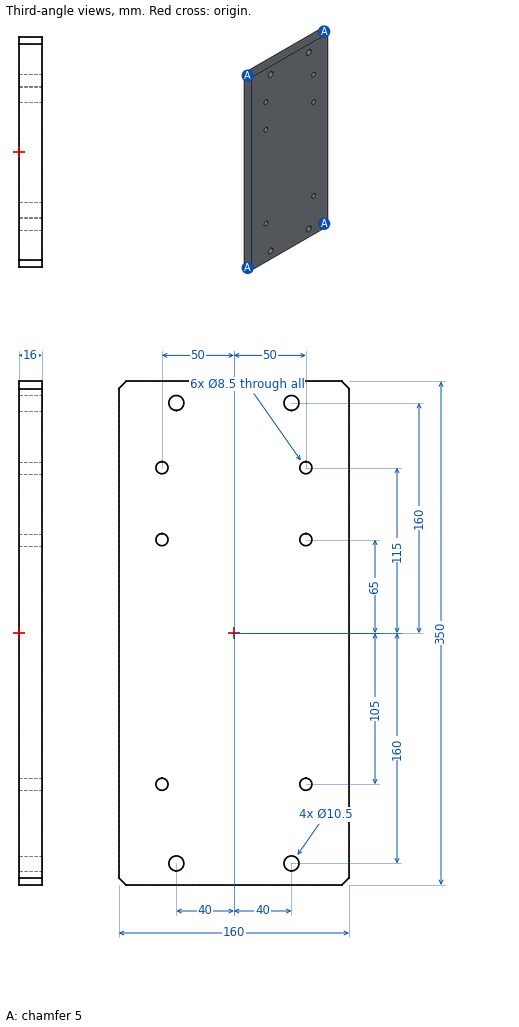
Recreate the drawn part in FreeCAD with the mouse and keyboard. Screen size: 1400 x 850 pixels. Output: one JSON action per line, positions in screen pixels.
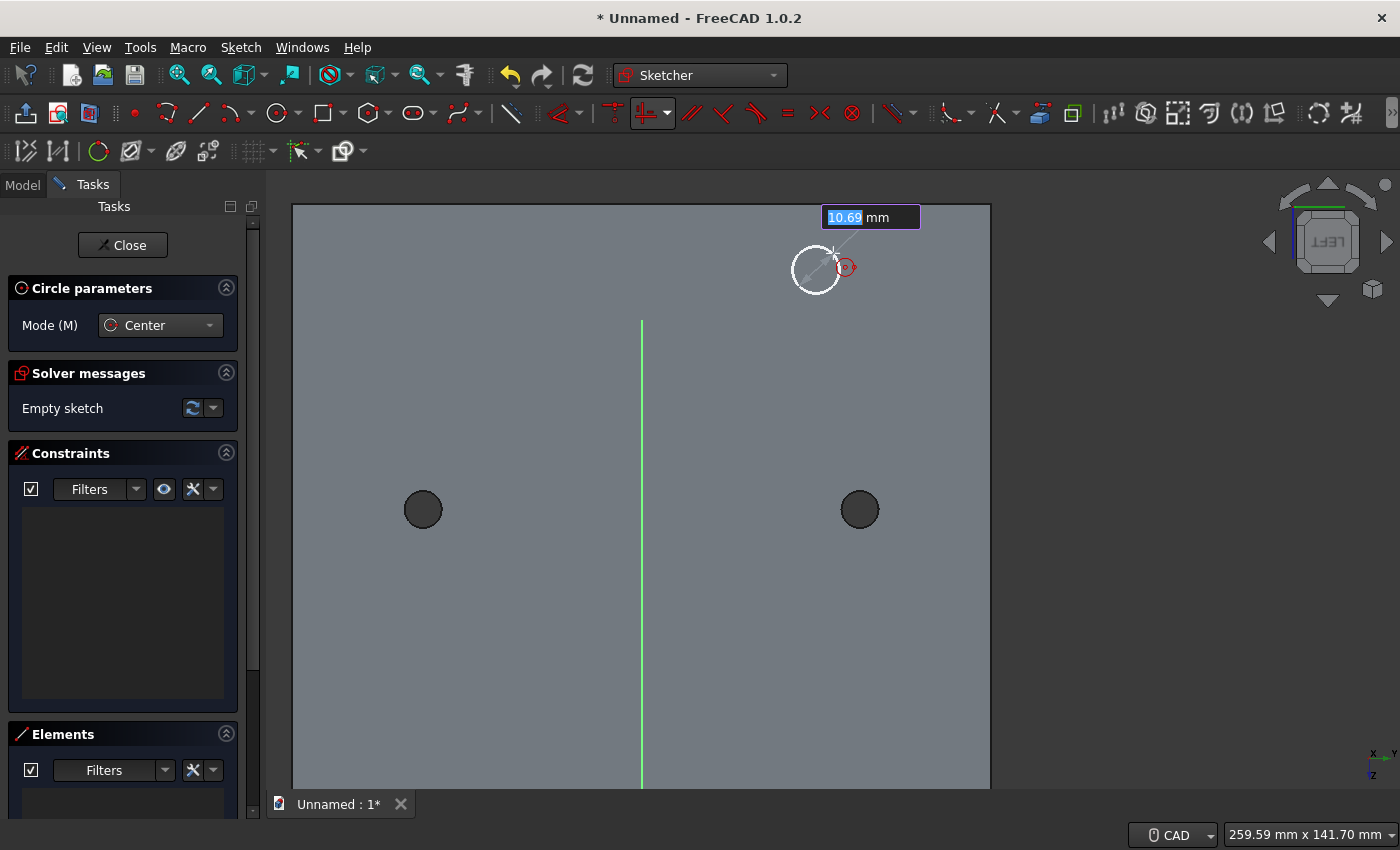
{"action": "type", "text": "10.5"}
{"action": "key", "text": "Return"}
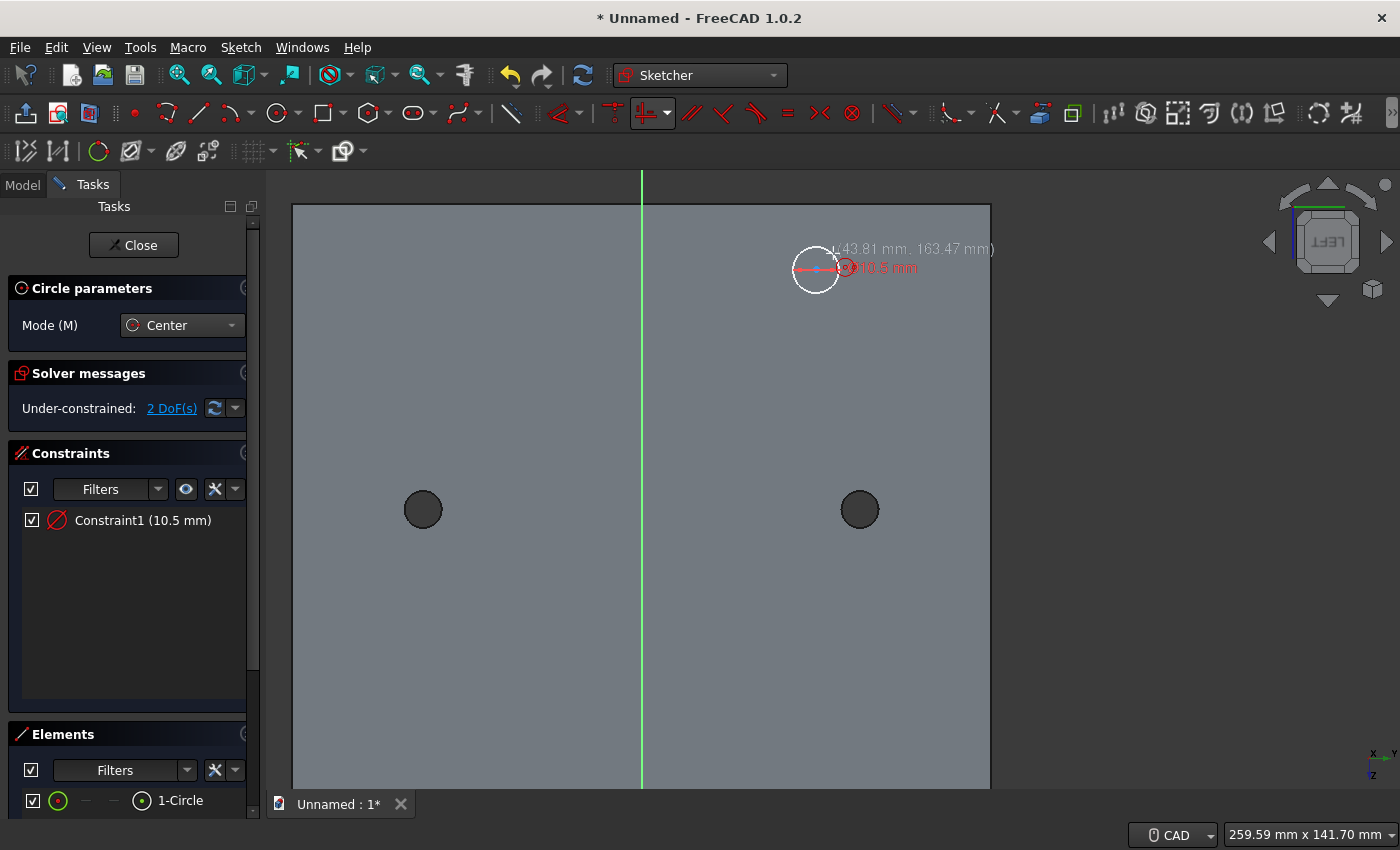
{"action": "left_click", "coordinate": [467, 269]}
{"action": "mouse_move", "coordinate": [483, 253]}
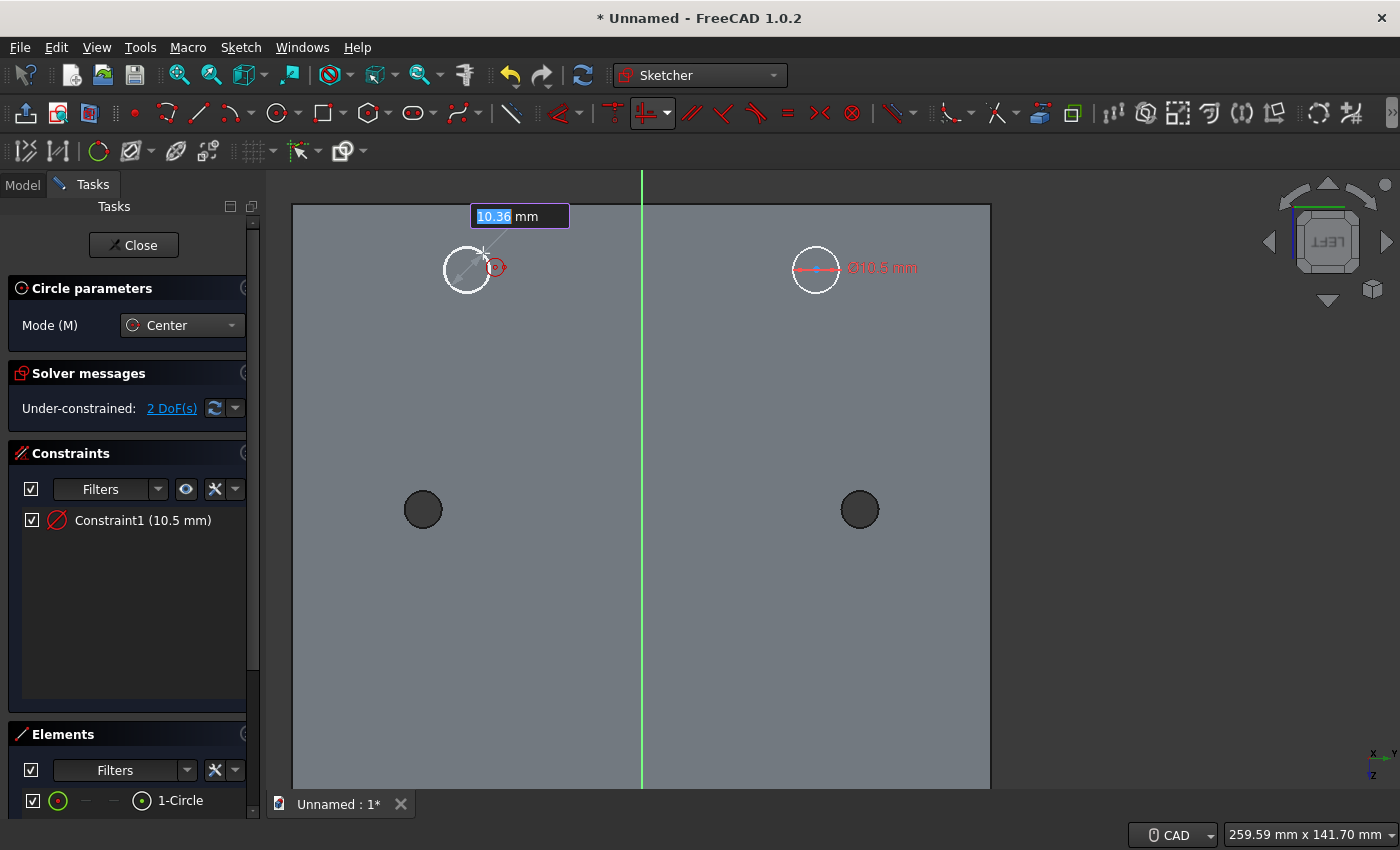
{"action": "type", "text": "10.5"}
{"action": "key", "text": "Return"}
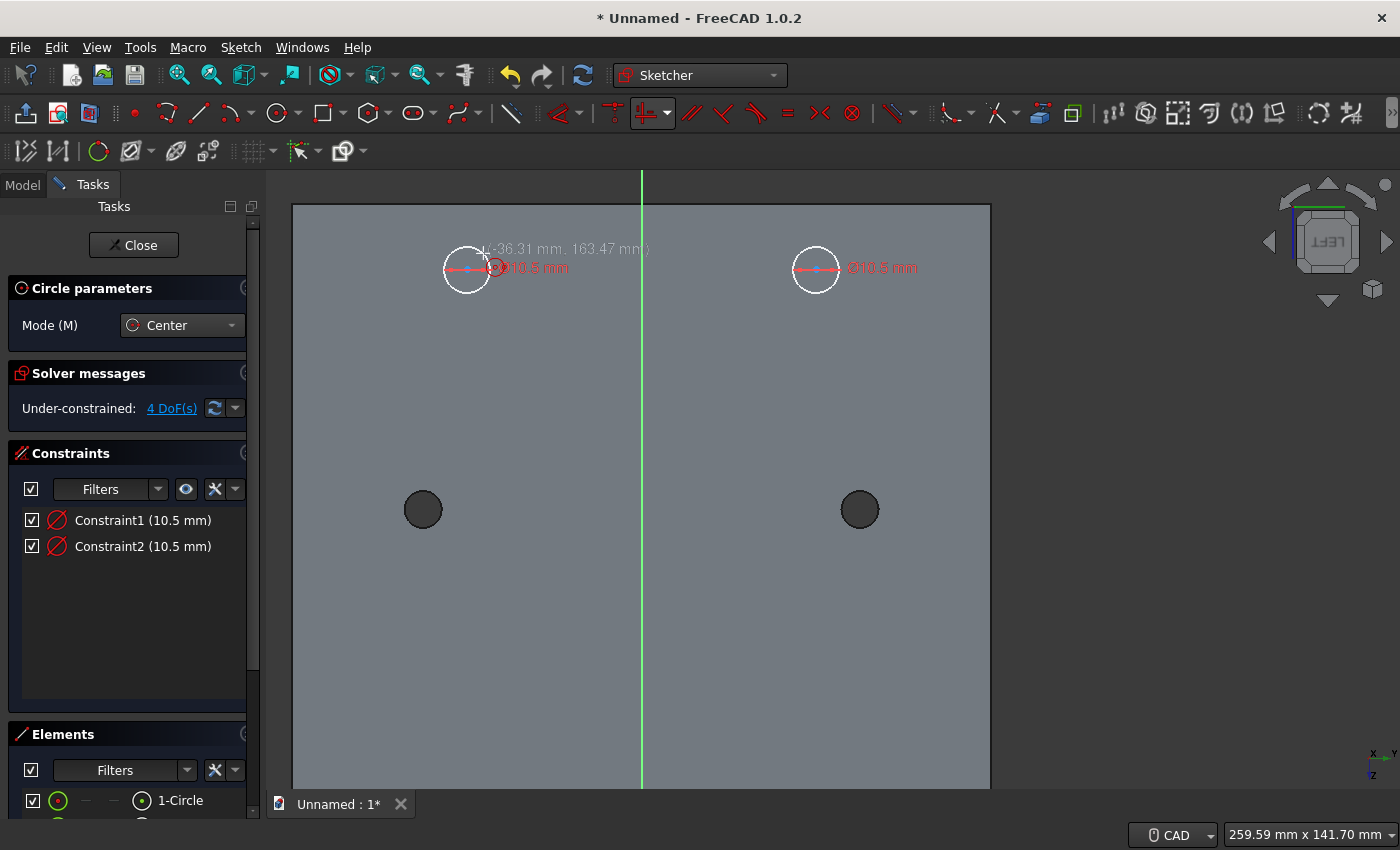
{"action": "scroll", "coordinate": [817, 269], "scroll_direction": "down", "scroll_amount": 6}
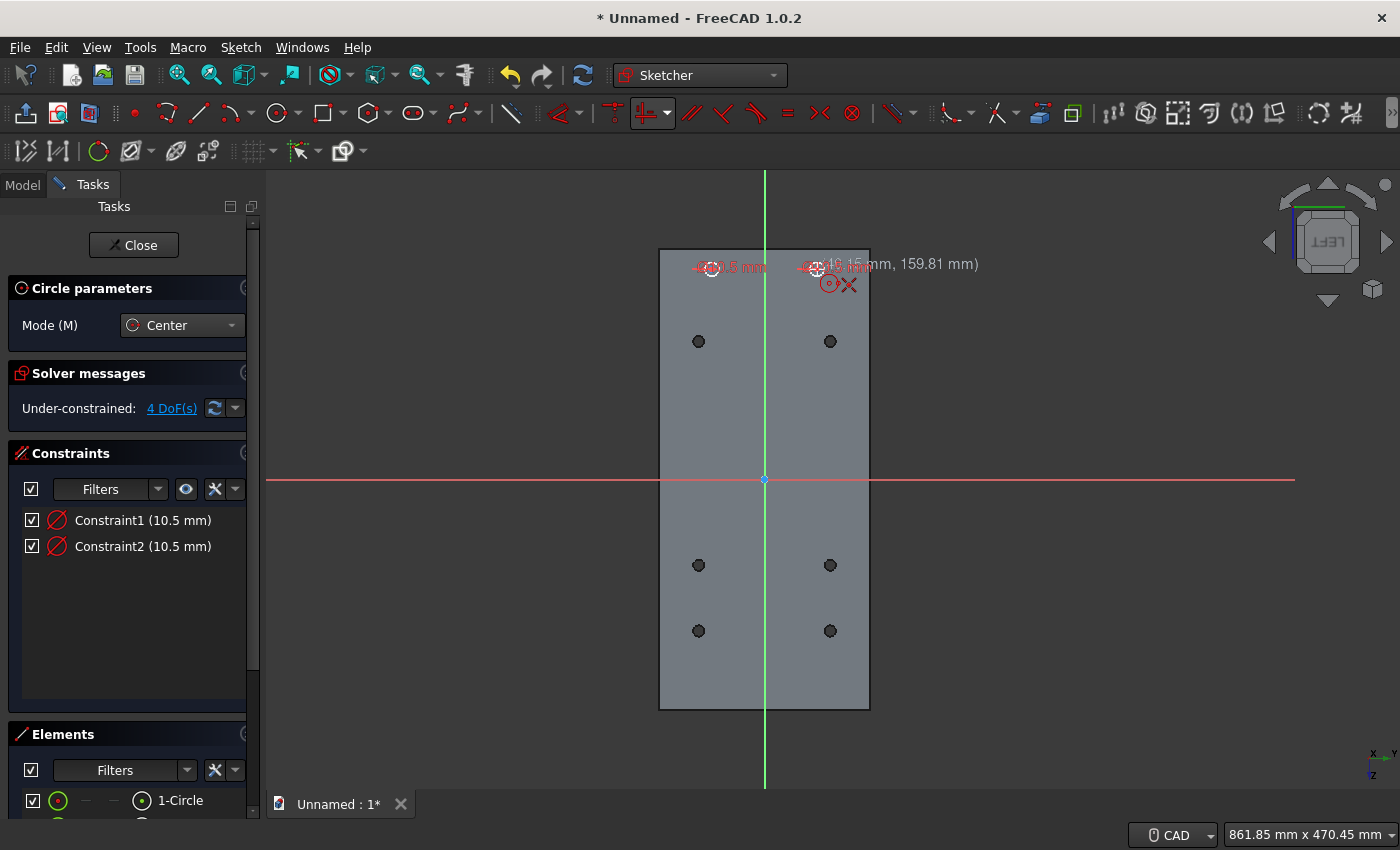
{"action": "scroll", "coordinate": [817, 690], "scroll_direction": "up", "scroll_amount": 6}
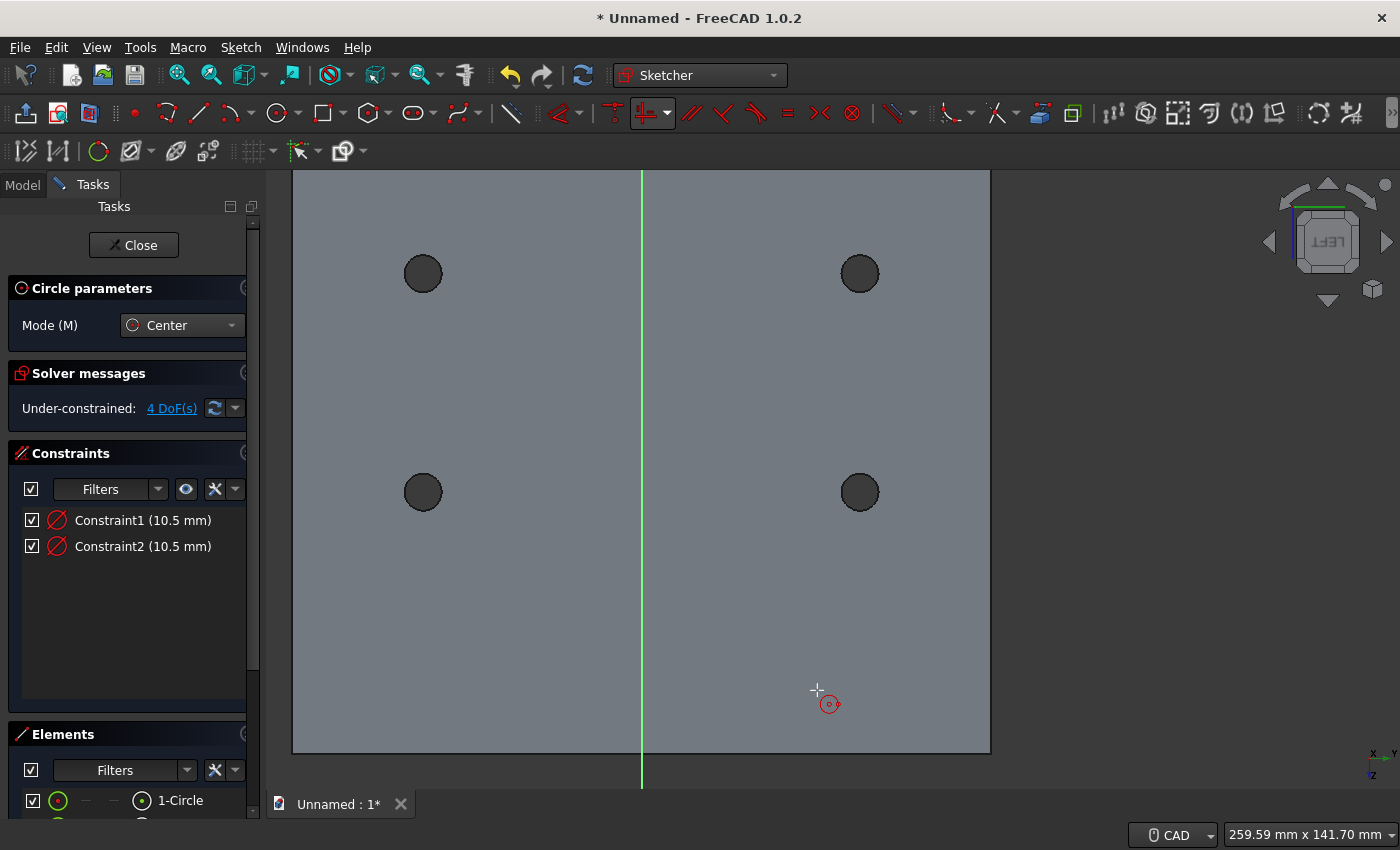
{"action": "left_click", "coordinate": [816, 689]}
{"action": "mouse_move", "coordinate": [833, 673]}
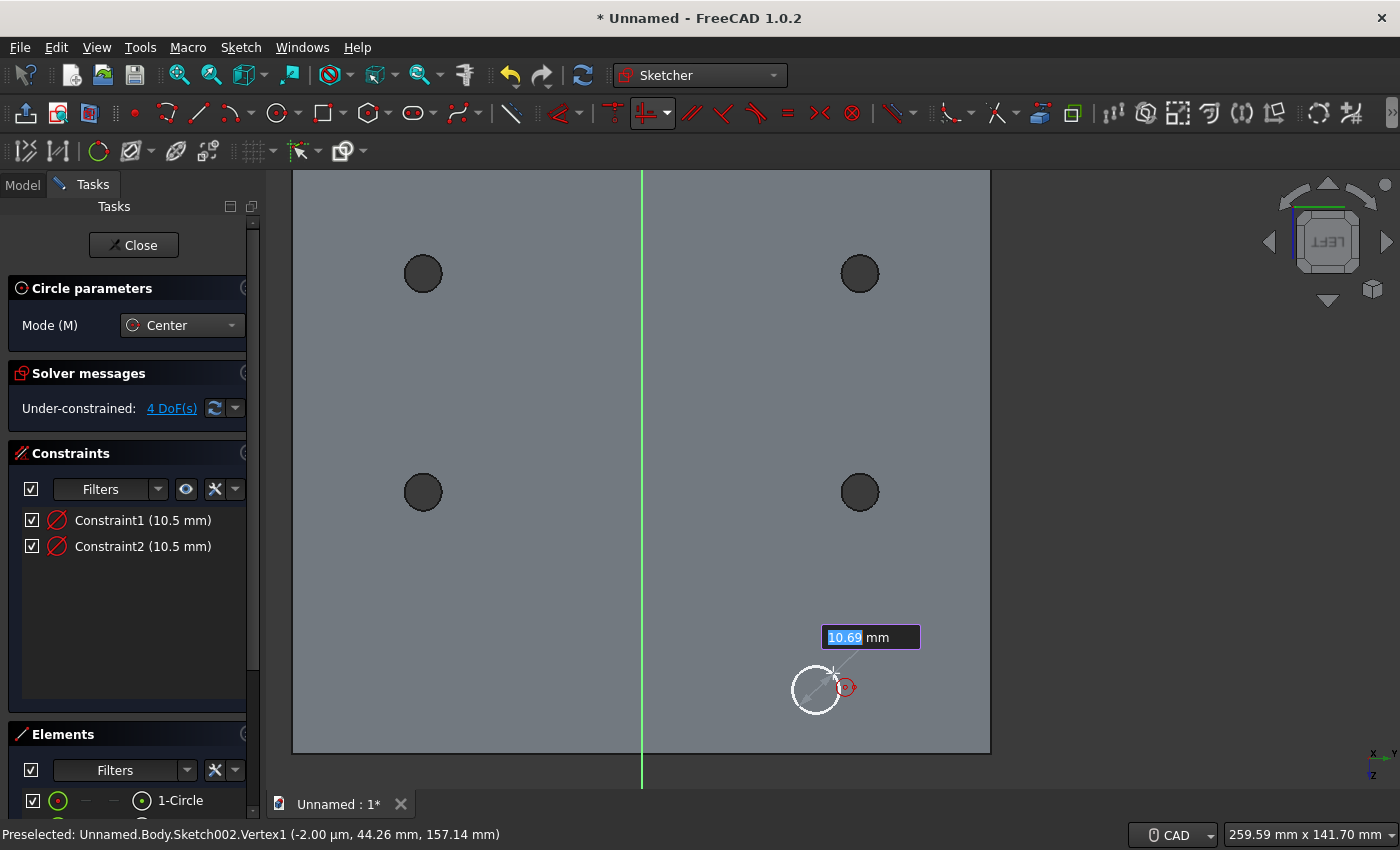
{"action": "type", "text": "10.5"}
{"action": "key", "text": "Return"}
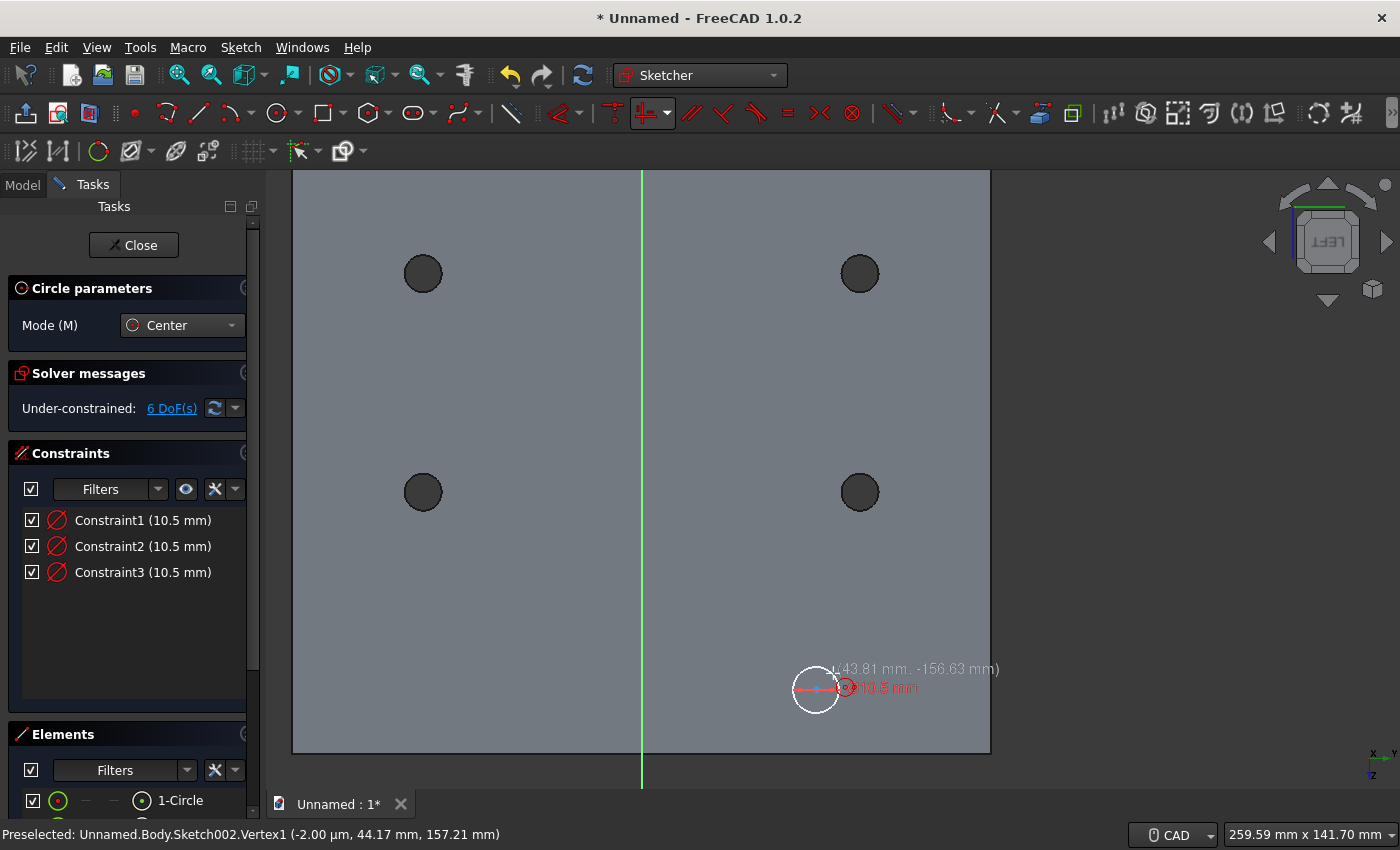
{"action": "left_click", "coordinate": [467, 689]}
{"action": "mouse_move", "coordinate": [483, 673]}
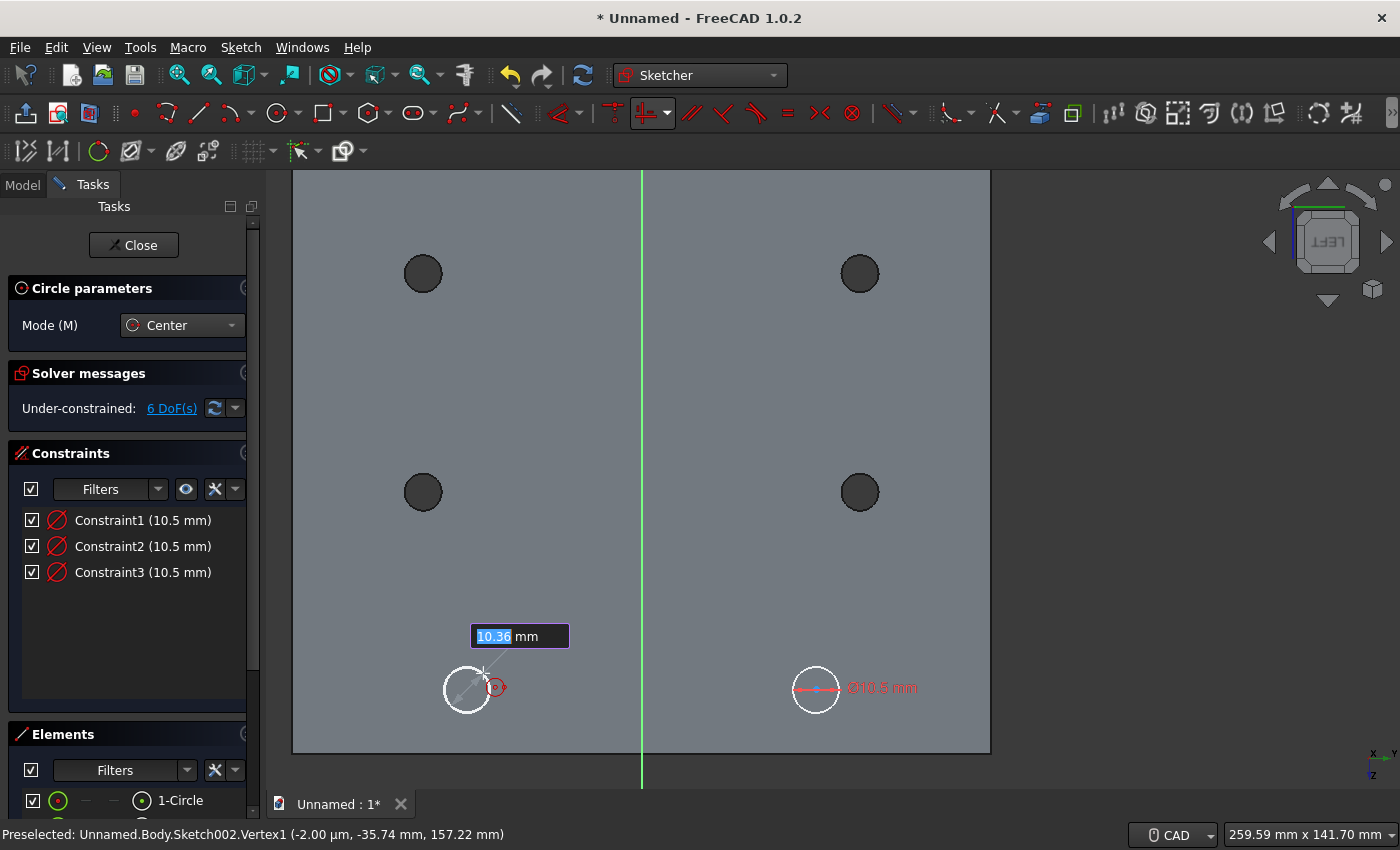
{"action": "type", "text": "10.5"}
{"action": "key", "text": "Return"}
{"action": "key", "text": "Escape"}